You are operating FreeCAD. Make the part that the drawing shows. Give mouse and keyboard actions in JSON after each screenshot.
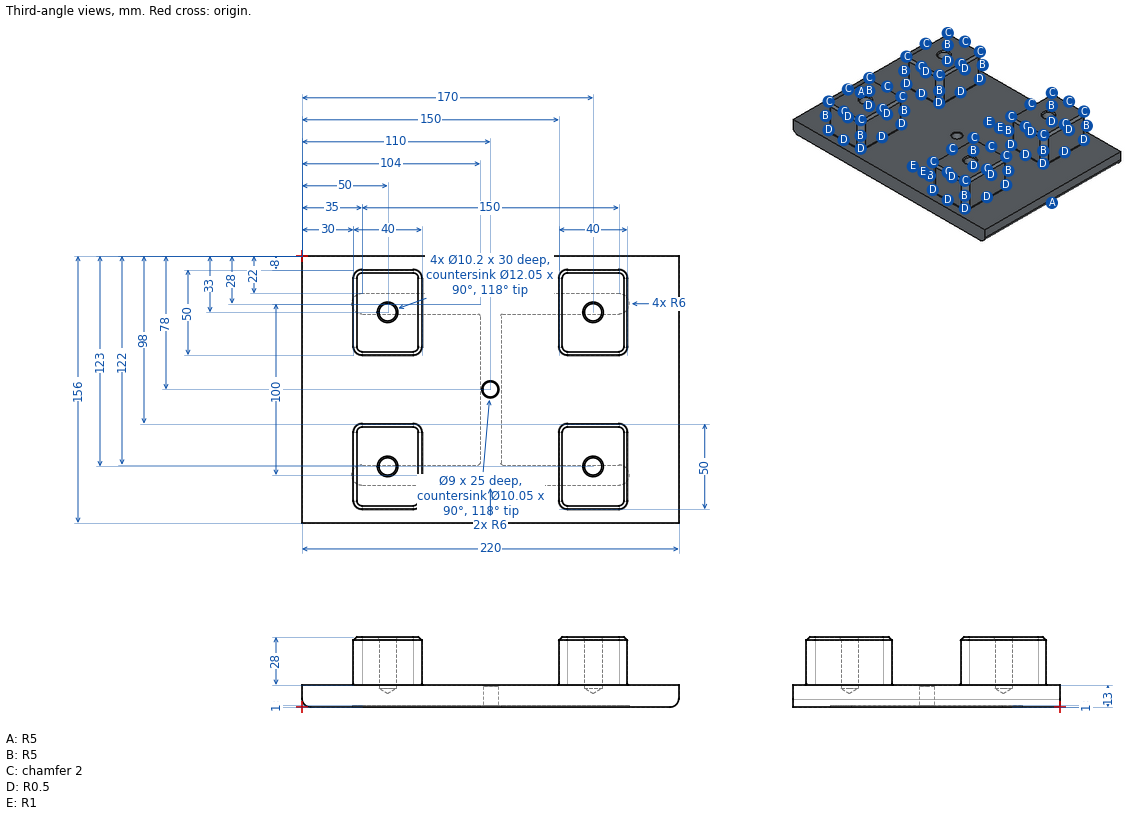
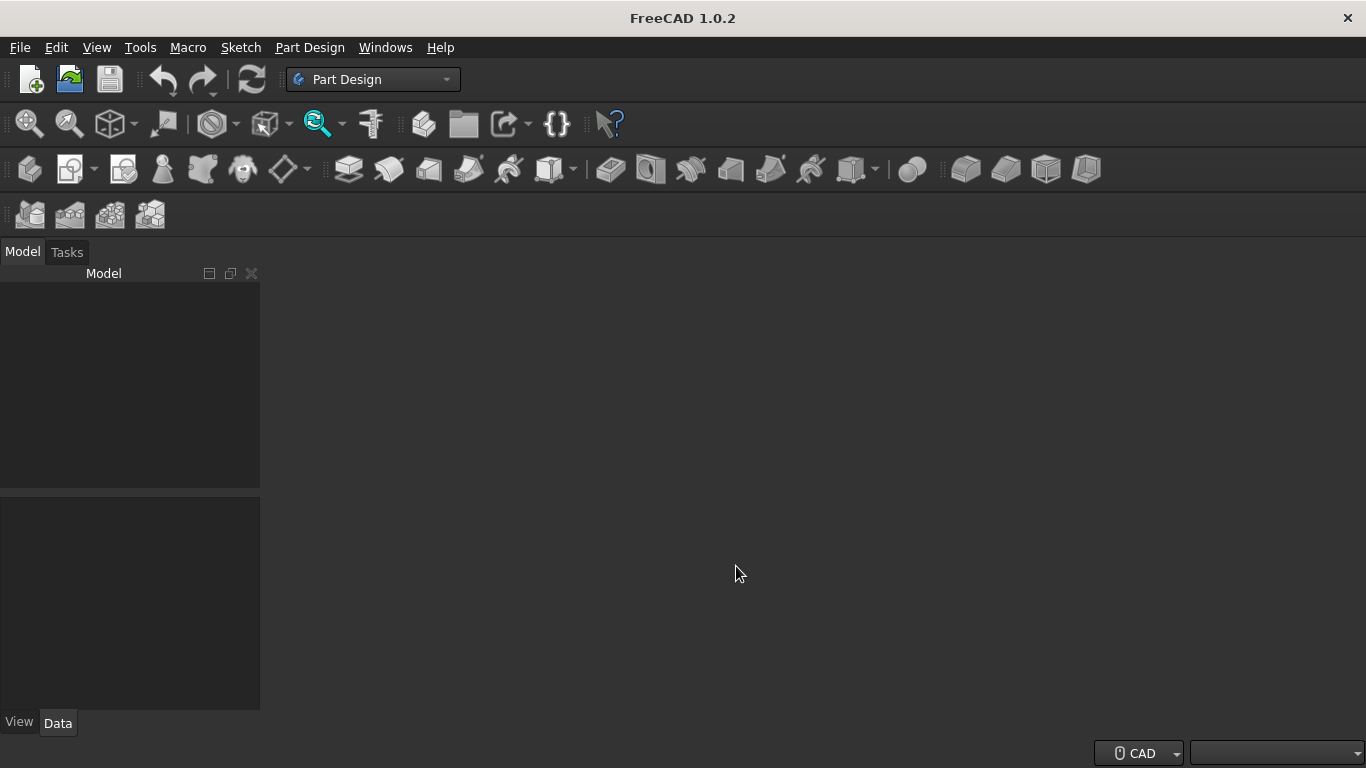
{"action": "key", "text": "ctrl+n"}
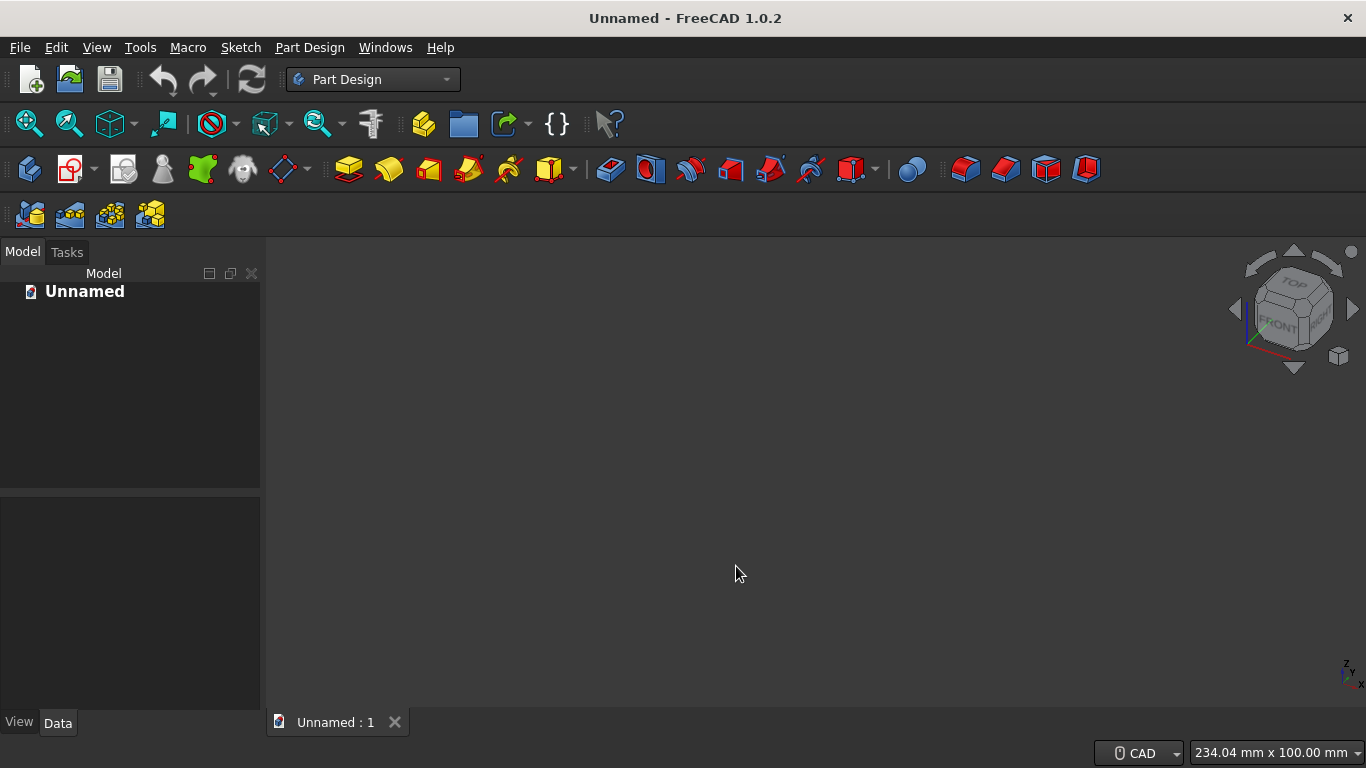
{"action": "left_click", "coordinate": [70, 170]}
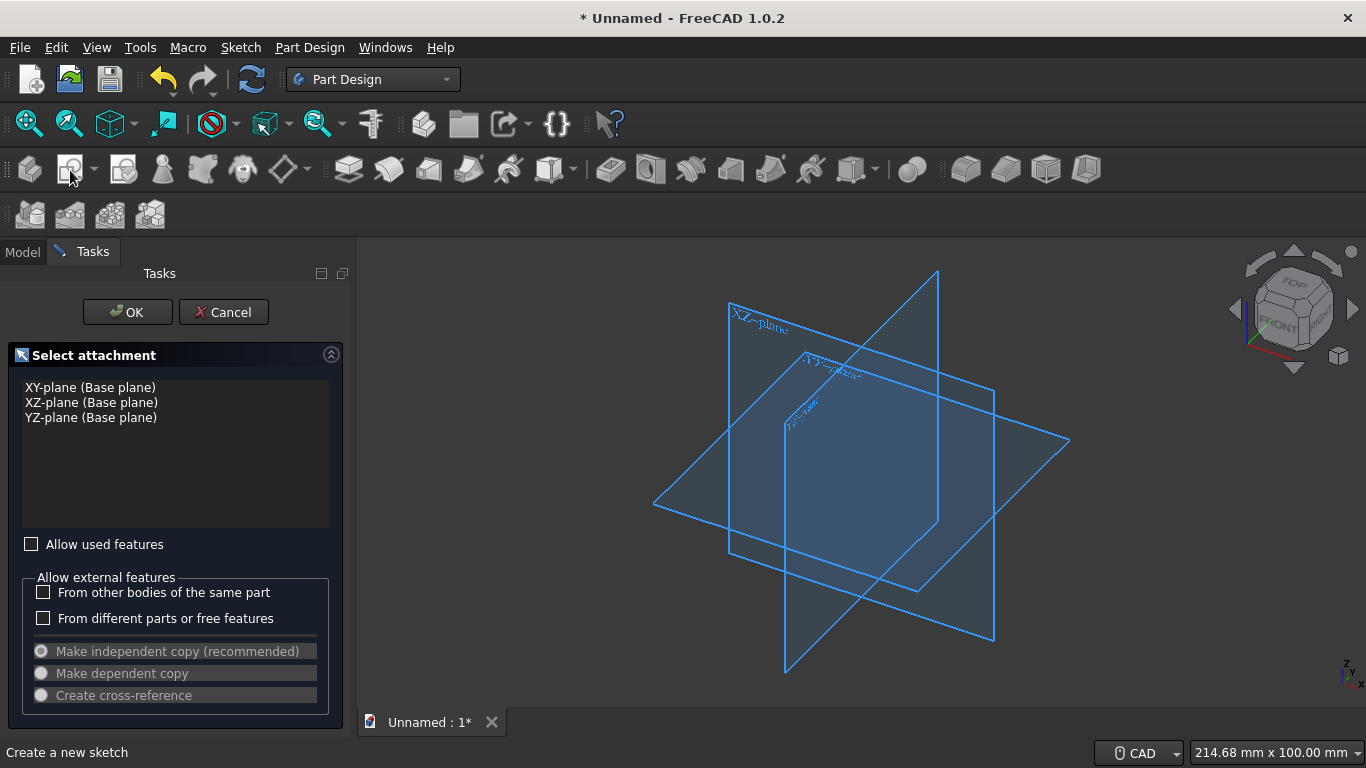
{"action": "left_click", "coordinate": [82, 388]}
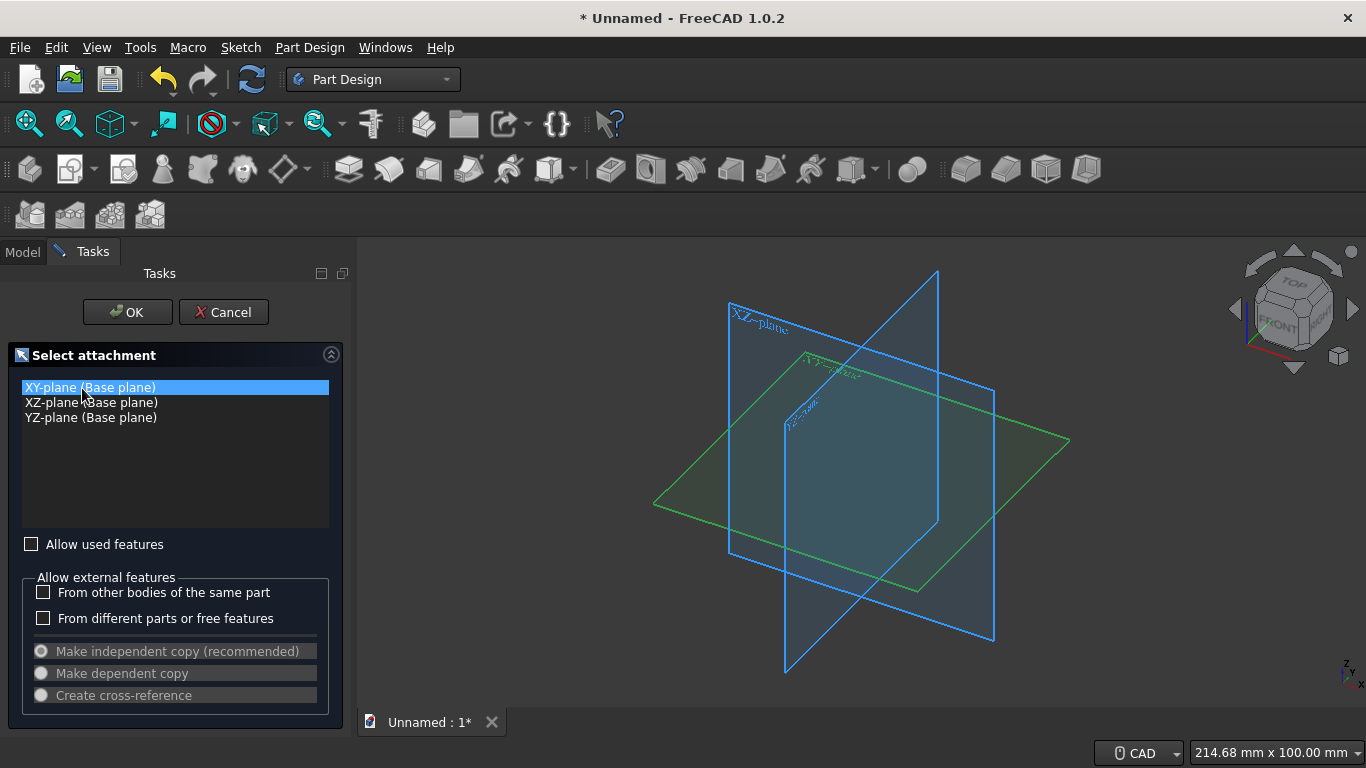
{"action": "left_click", "coordinate": [128, 312]}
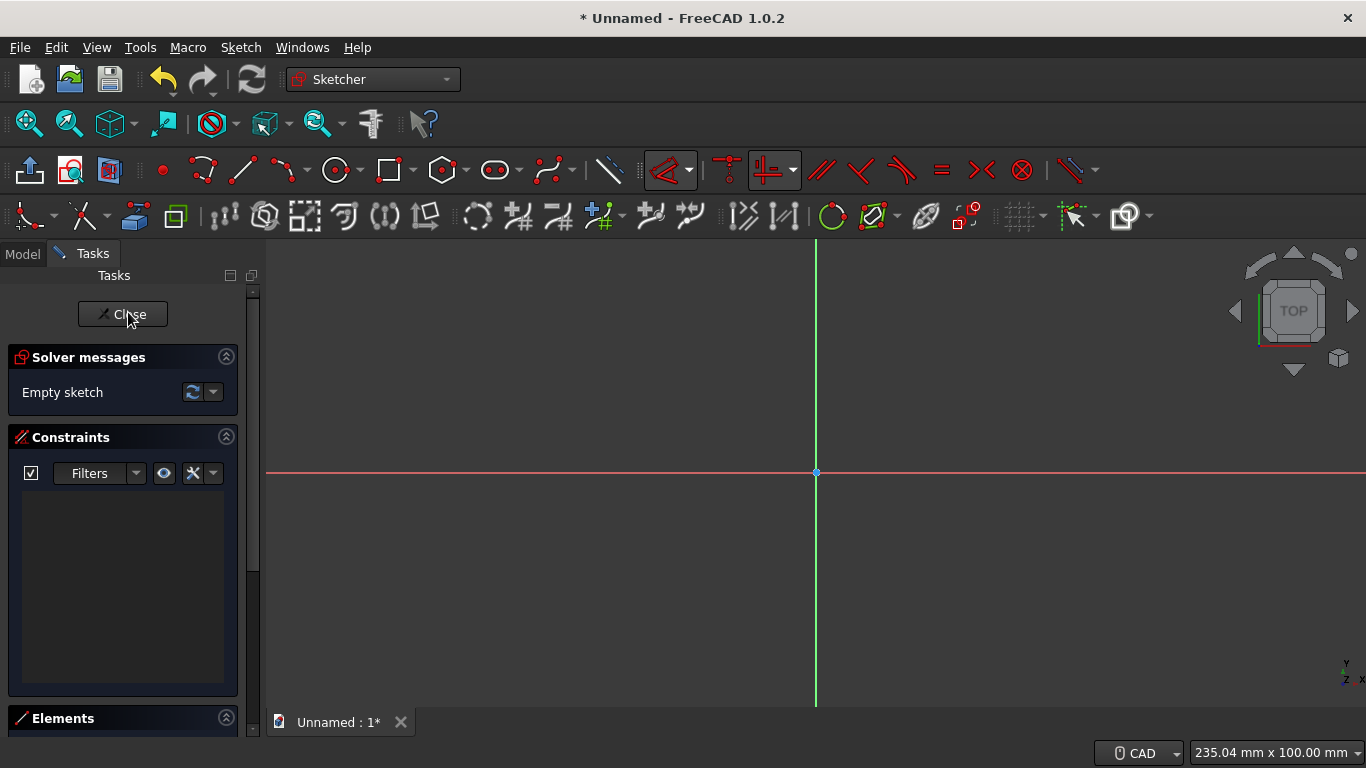
{"action": "scroll", "coordinate": [408, 267], "scroll_direction": "down", "scroll_amount": 5}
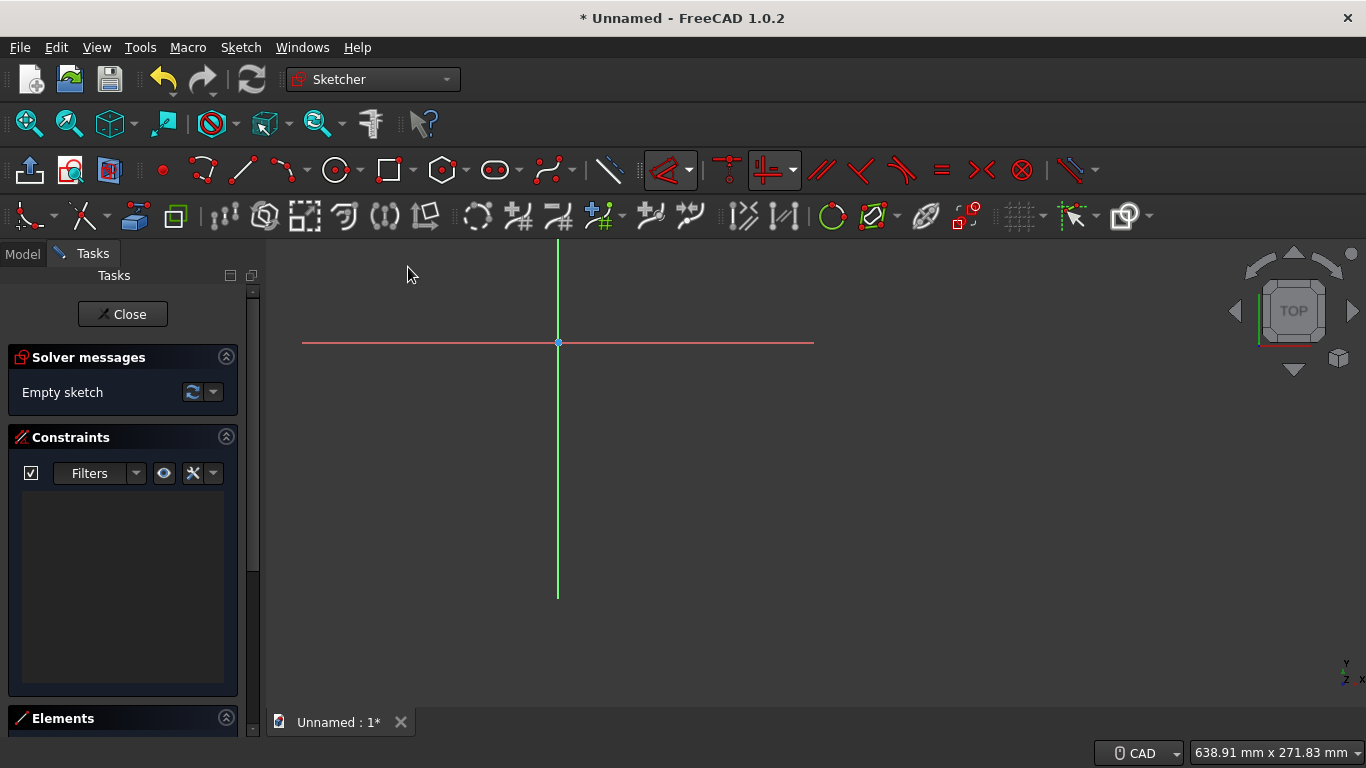
{"action": "key", "text": "g r"}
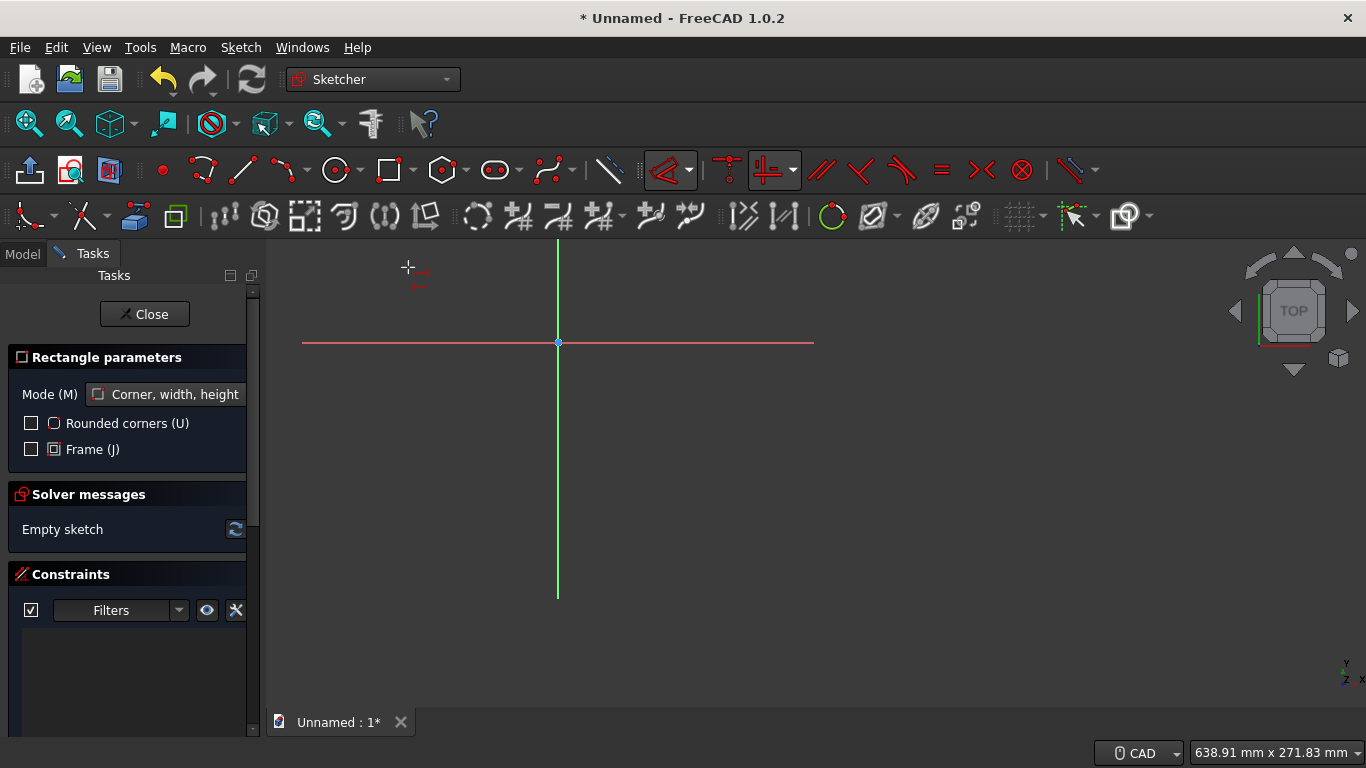
{"action": "left_click", "coordinate": [558, 343]}
{"action": "left_click", "coordinate": [937, 611]}
{"action": "key", "text": "Escape"}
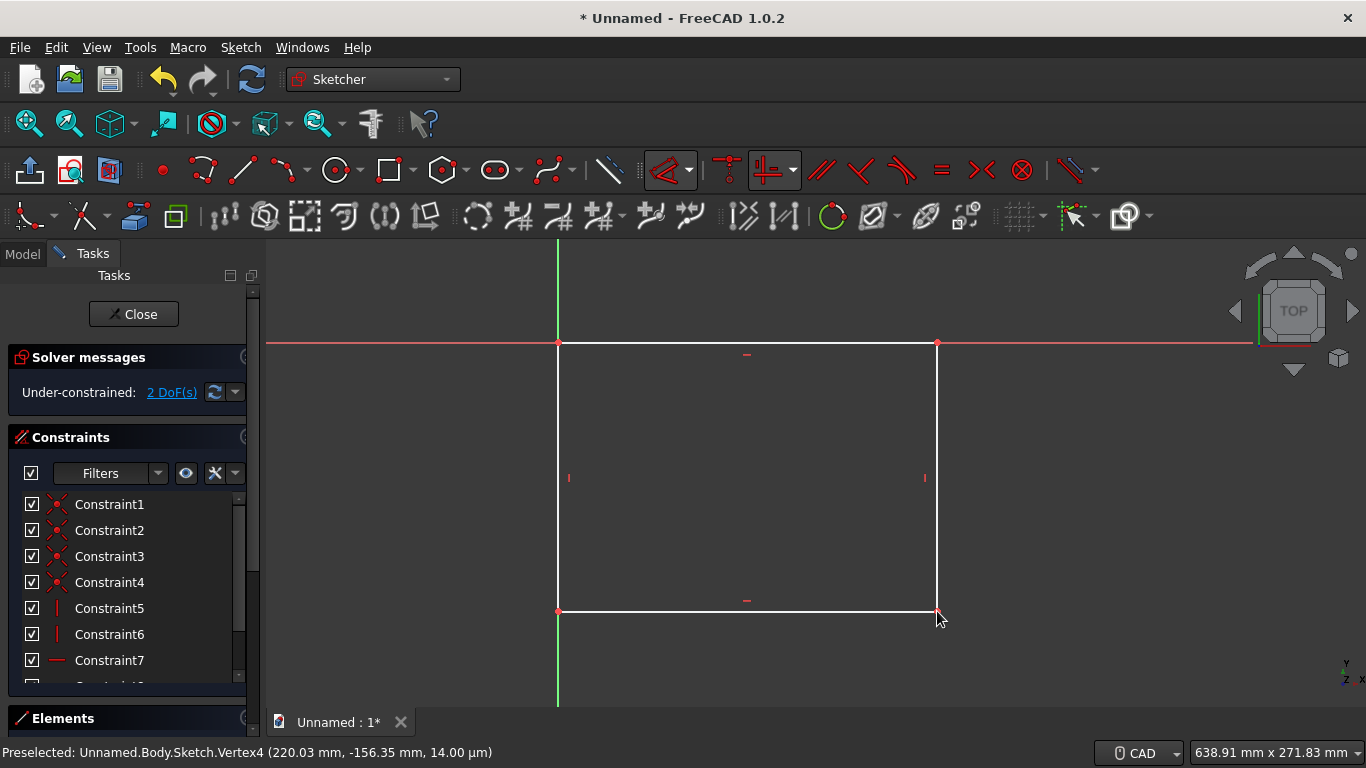
{"action": "left_click", "coordinate": [664, 170]}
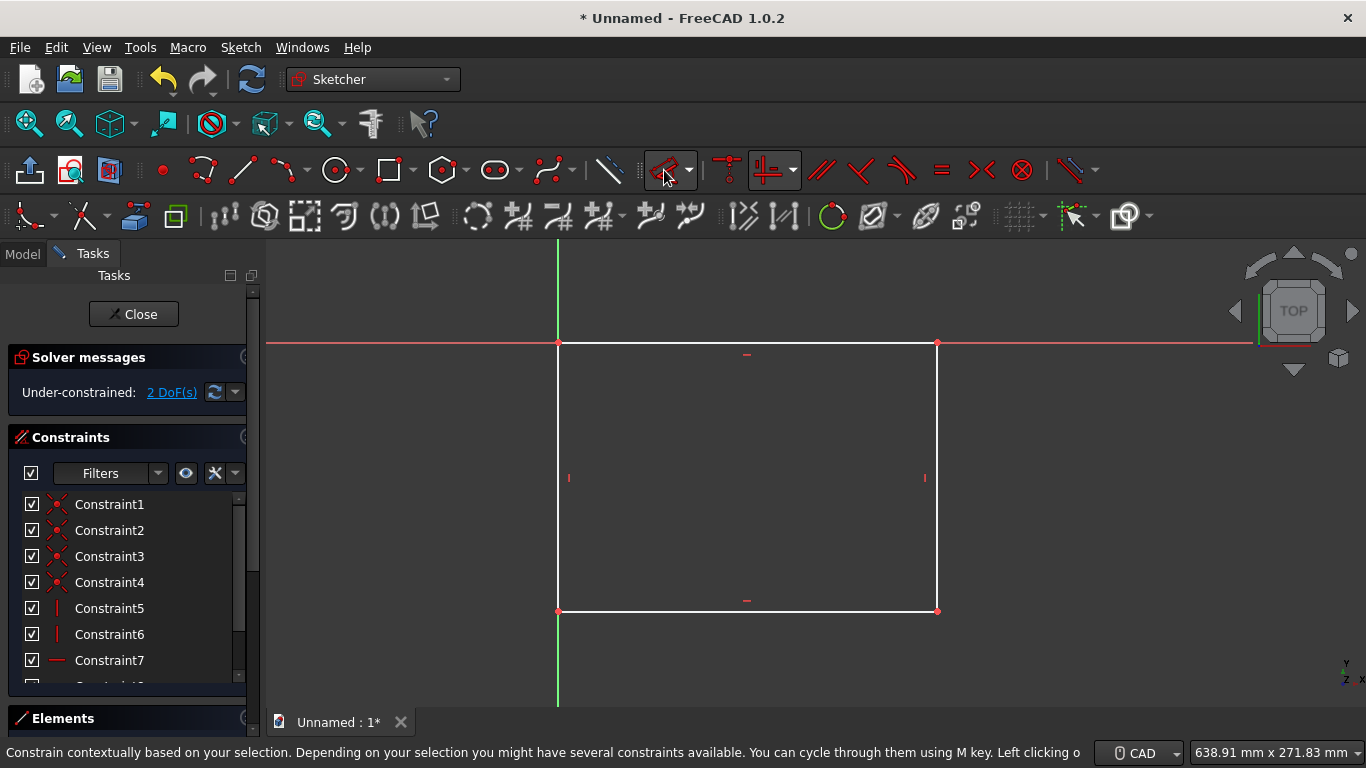
{"action": "left_click", "coordinate": [558, 424]}
{"action": "left_click", "coordinate": [524, 477]}